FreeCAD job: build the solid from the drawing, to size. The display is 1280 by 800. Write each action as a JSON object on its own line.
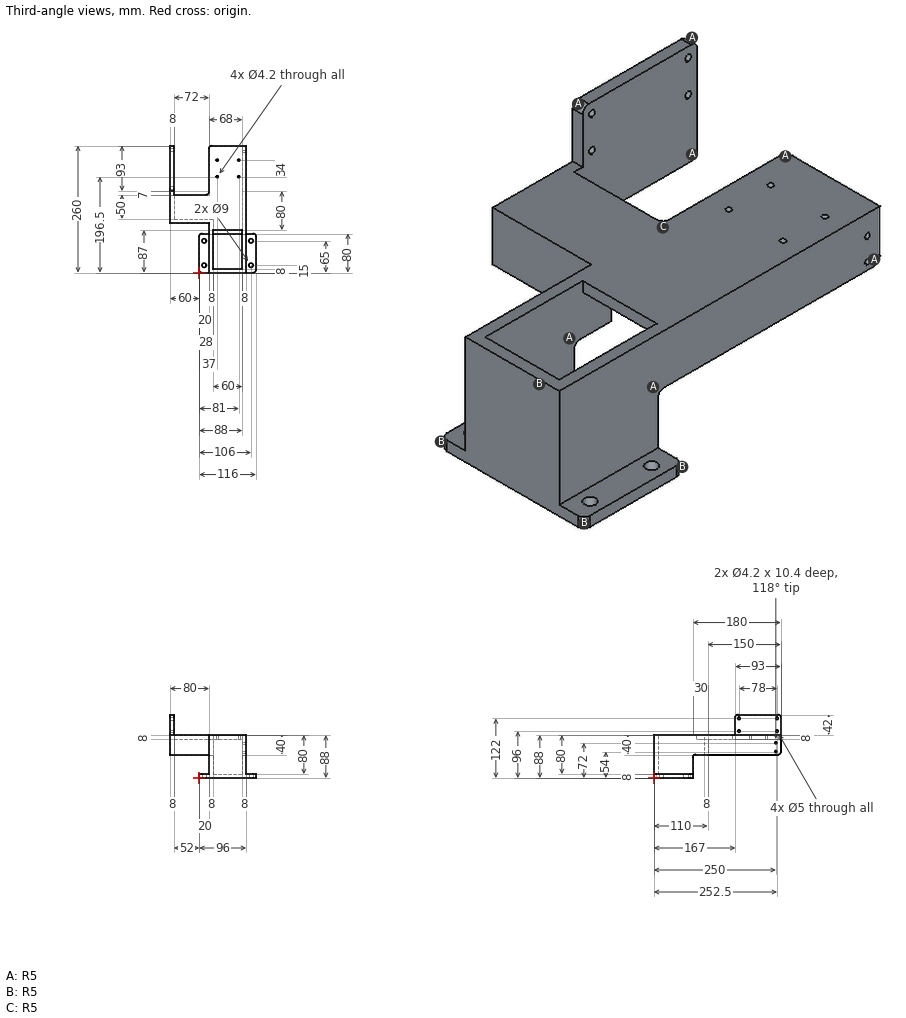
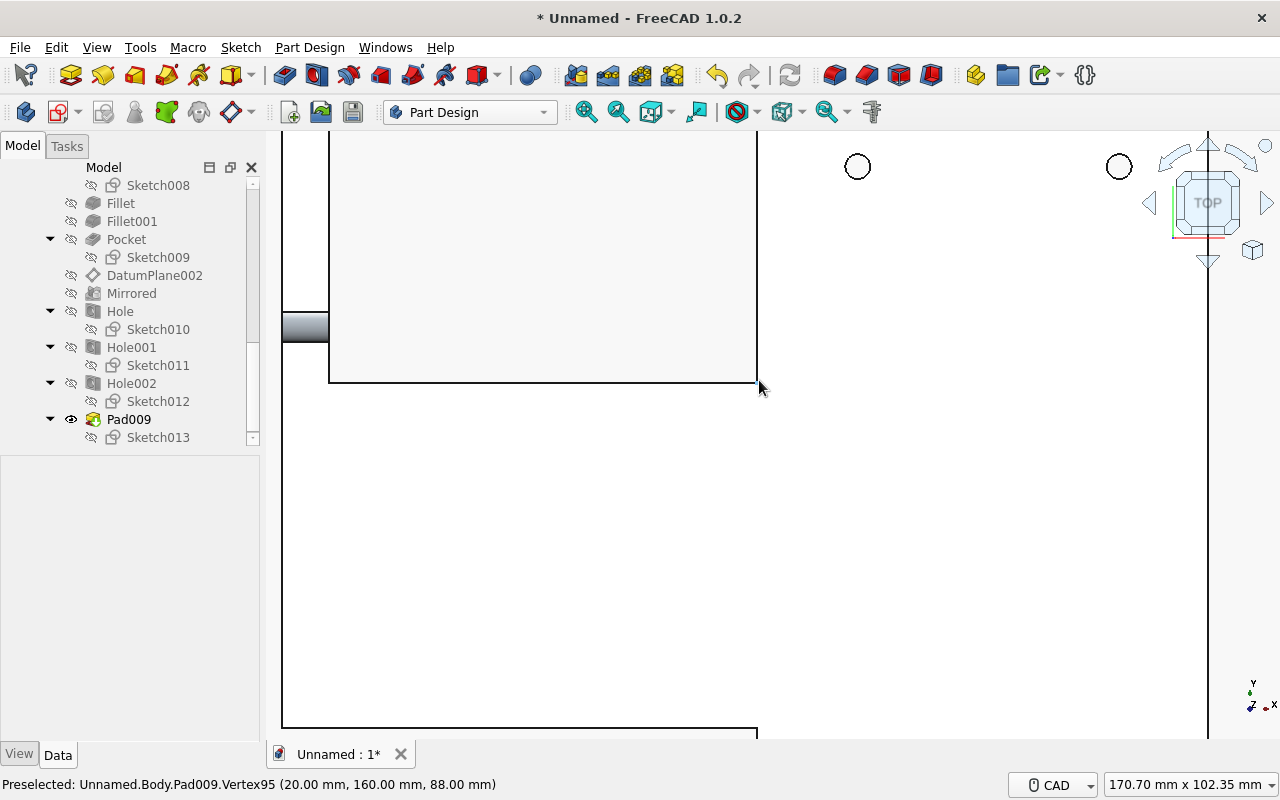
{"action": "left_click", "coordinate": [588, 112]}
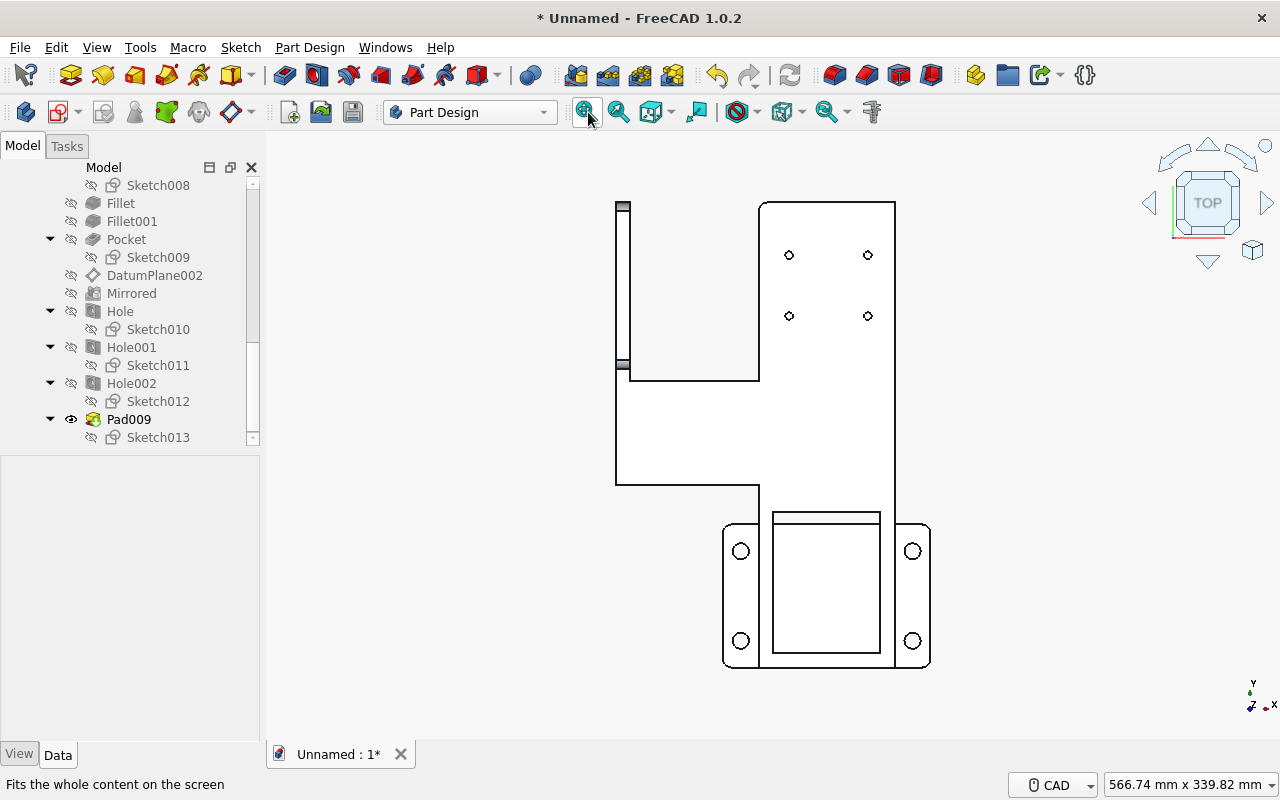
{"action": "key", "text": "0"}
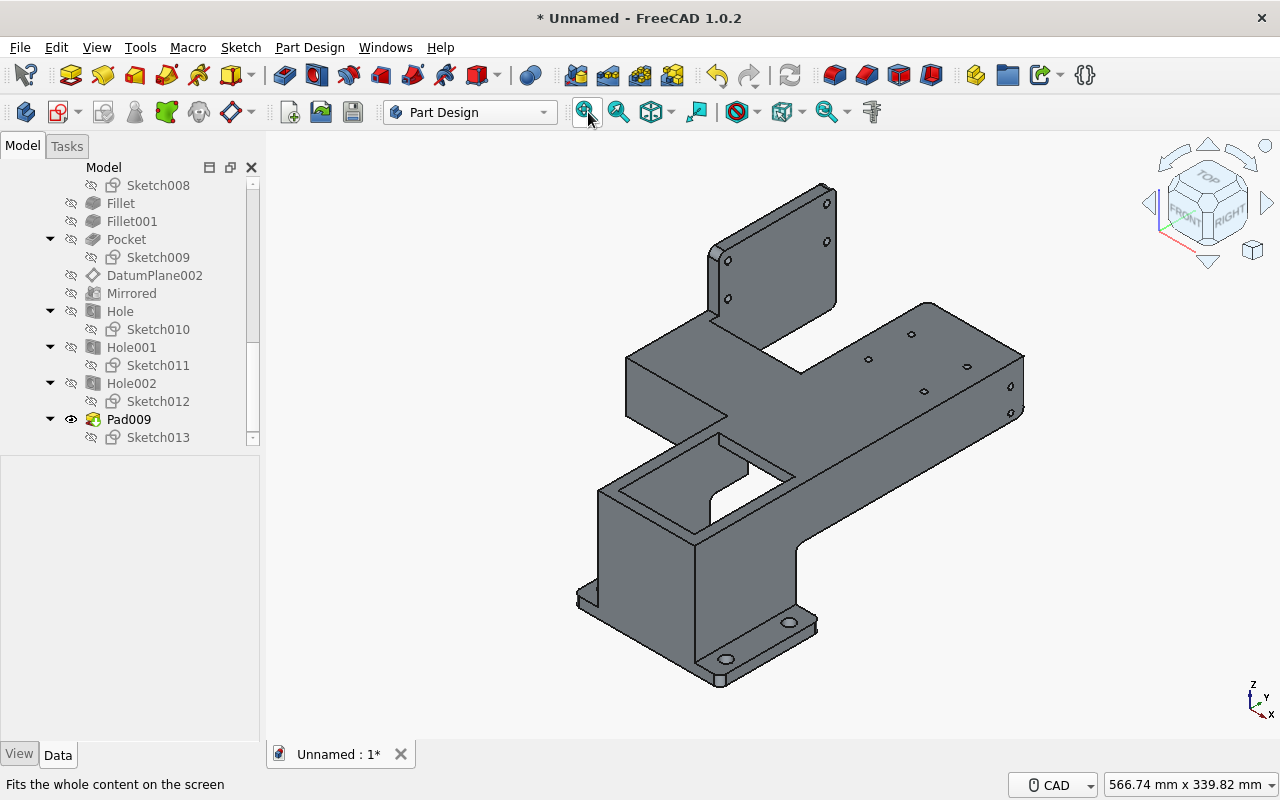
{"action": "scroll", "coordinate": [801, 378], "scroll_direction": "up", "scroll_amount": 6}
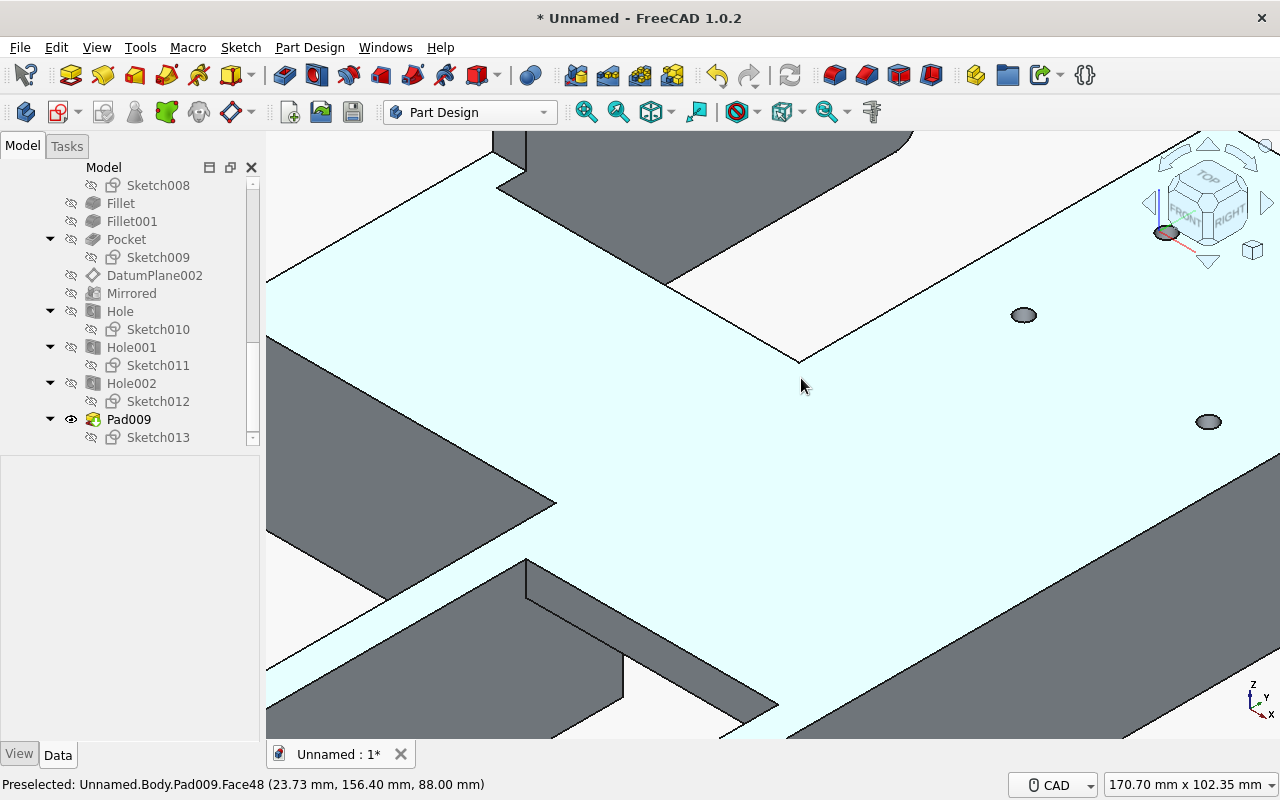
{"action": "left_click", "coordinate": [588, 112]}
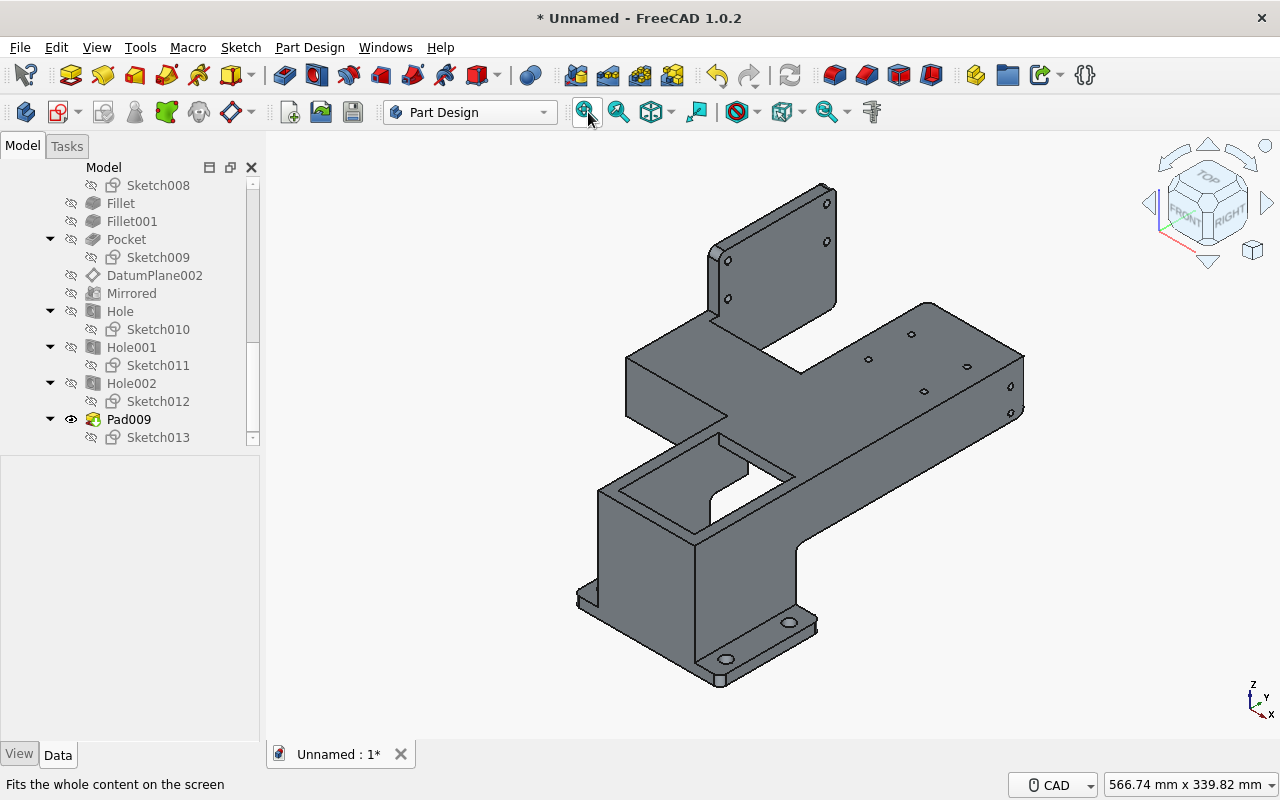
{"action": "key", "text": "1"}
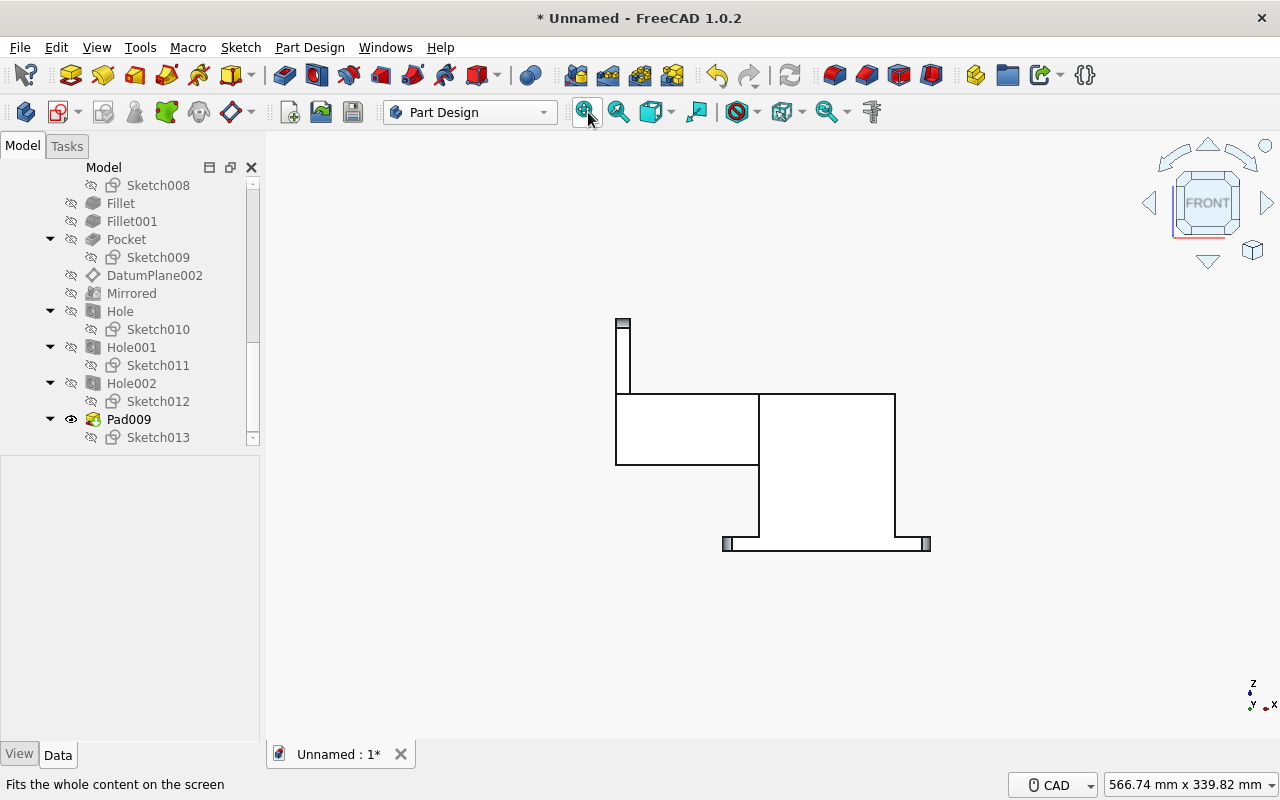
{"action": "left_click", "coordinate": [588, 112]}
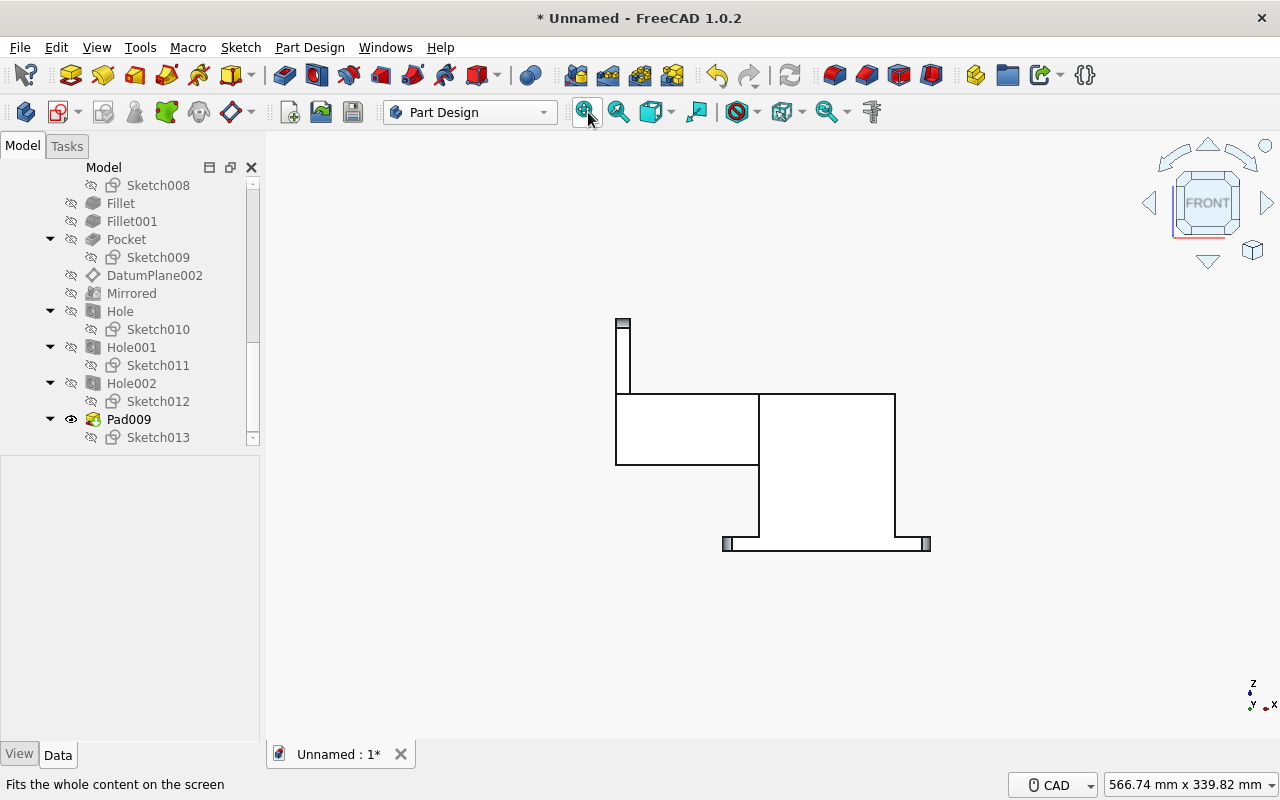
{"action": "scroll", "coordinate": [759, 400], "scroll_direction": "up", "scroll_amount": 6}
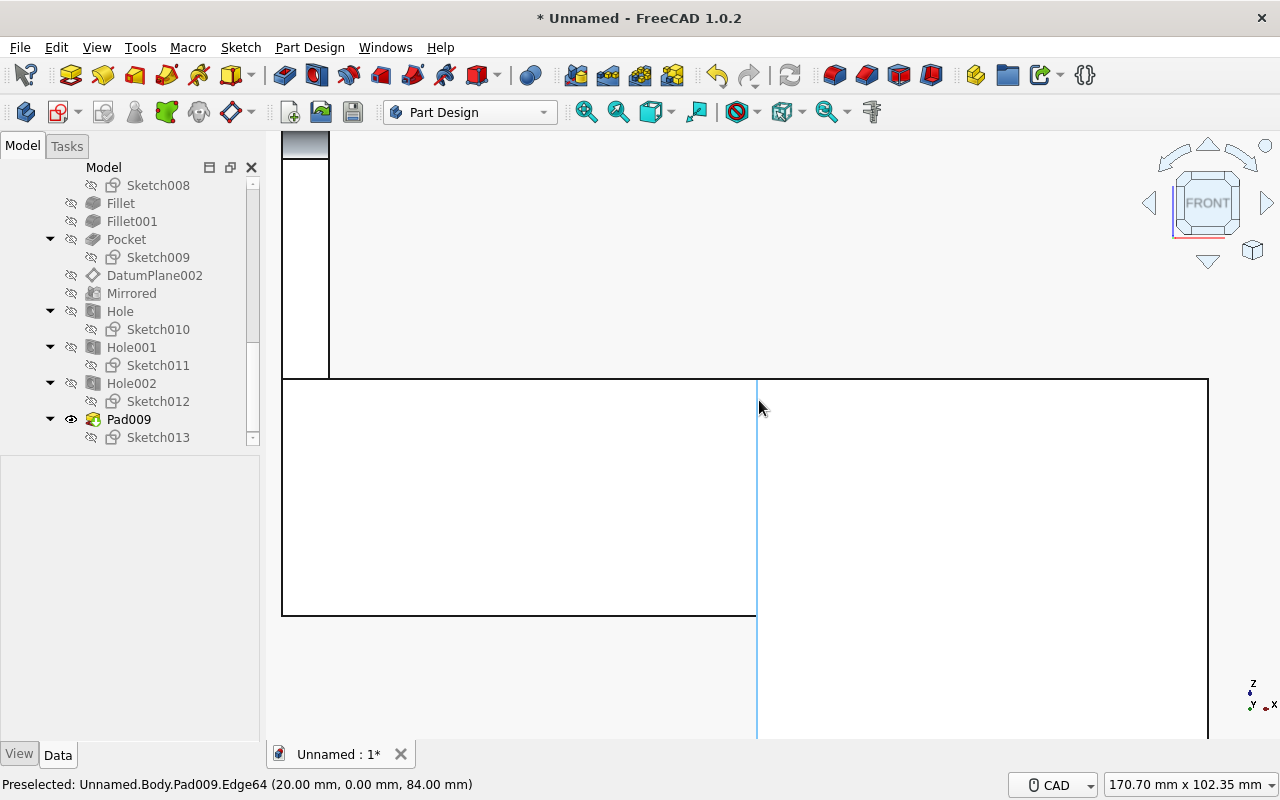
{"action": "left_click", "coordinate": [588, 112]}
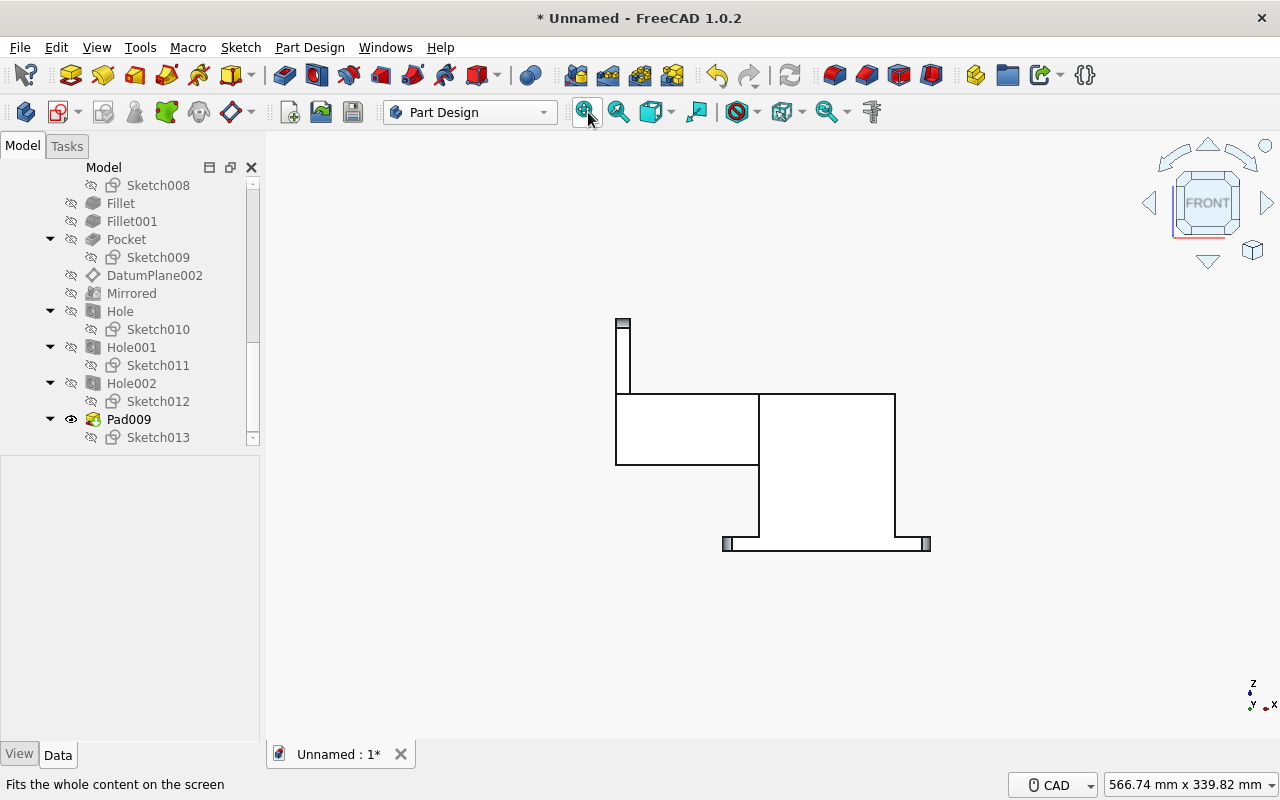
{"action": "key", "text": "3"}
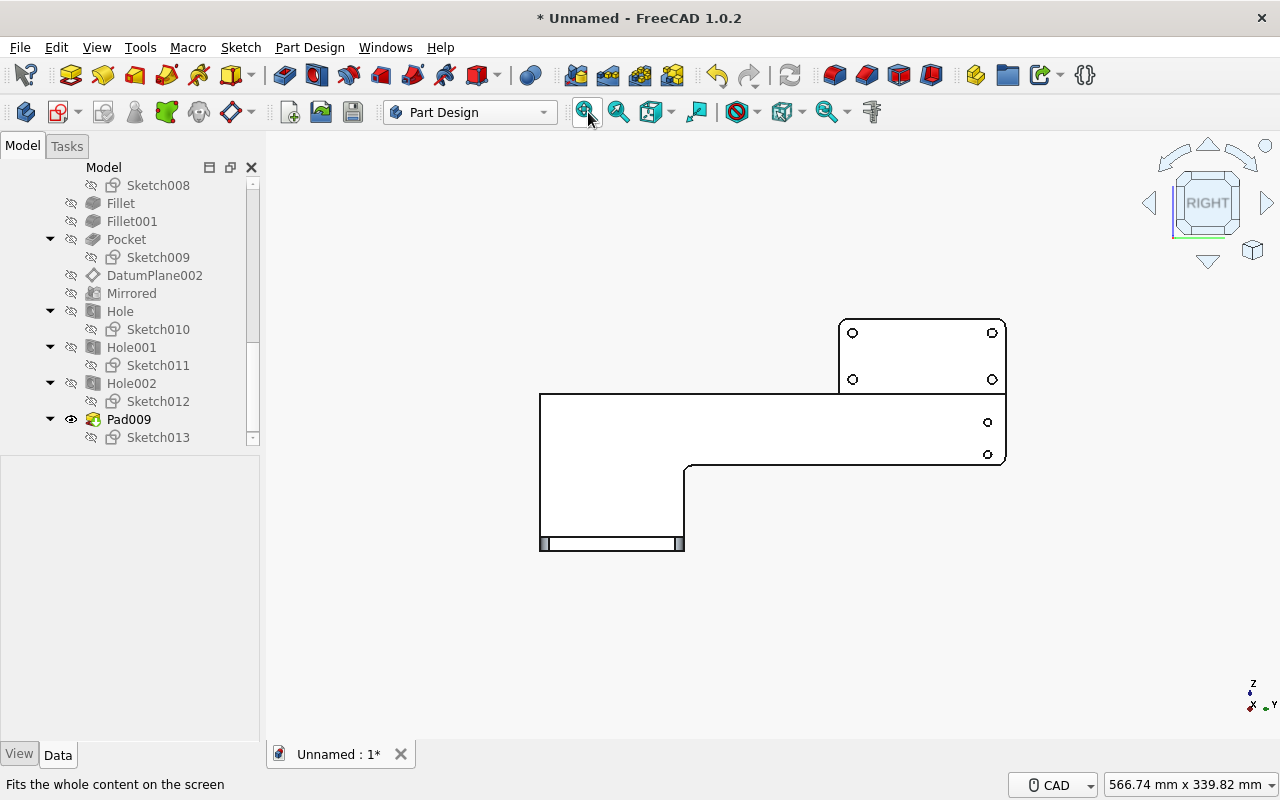
{"action": "scroll", "coordinate": [827, 400], "scroll_direction": "up", "scroll_amount": 6}